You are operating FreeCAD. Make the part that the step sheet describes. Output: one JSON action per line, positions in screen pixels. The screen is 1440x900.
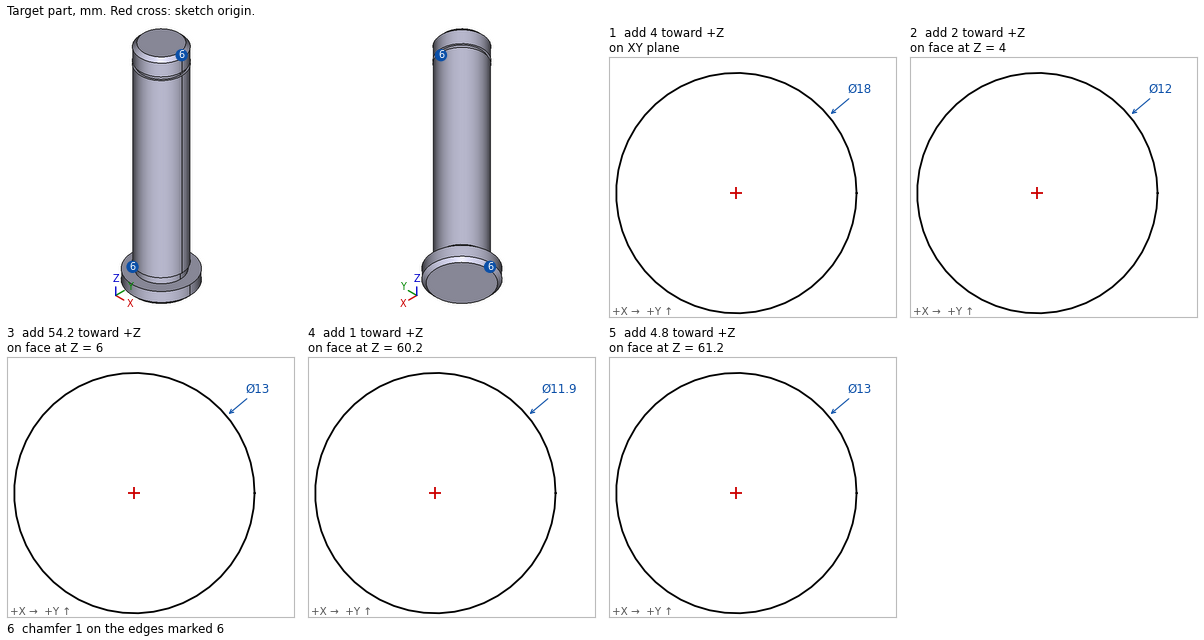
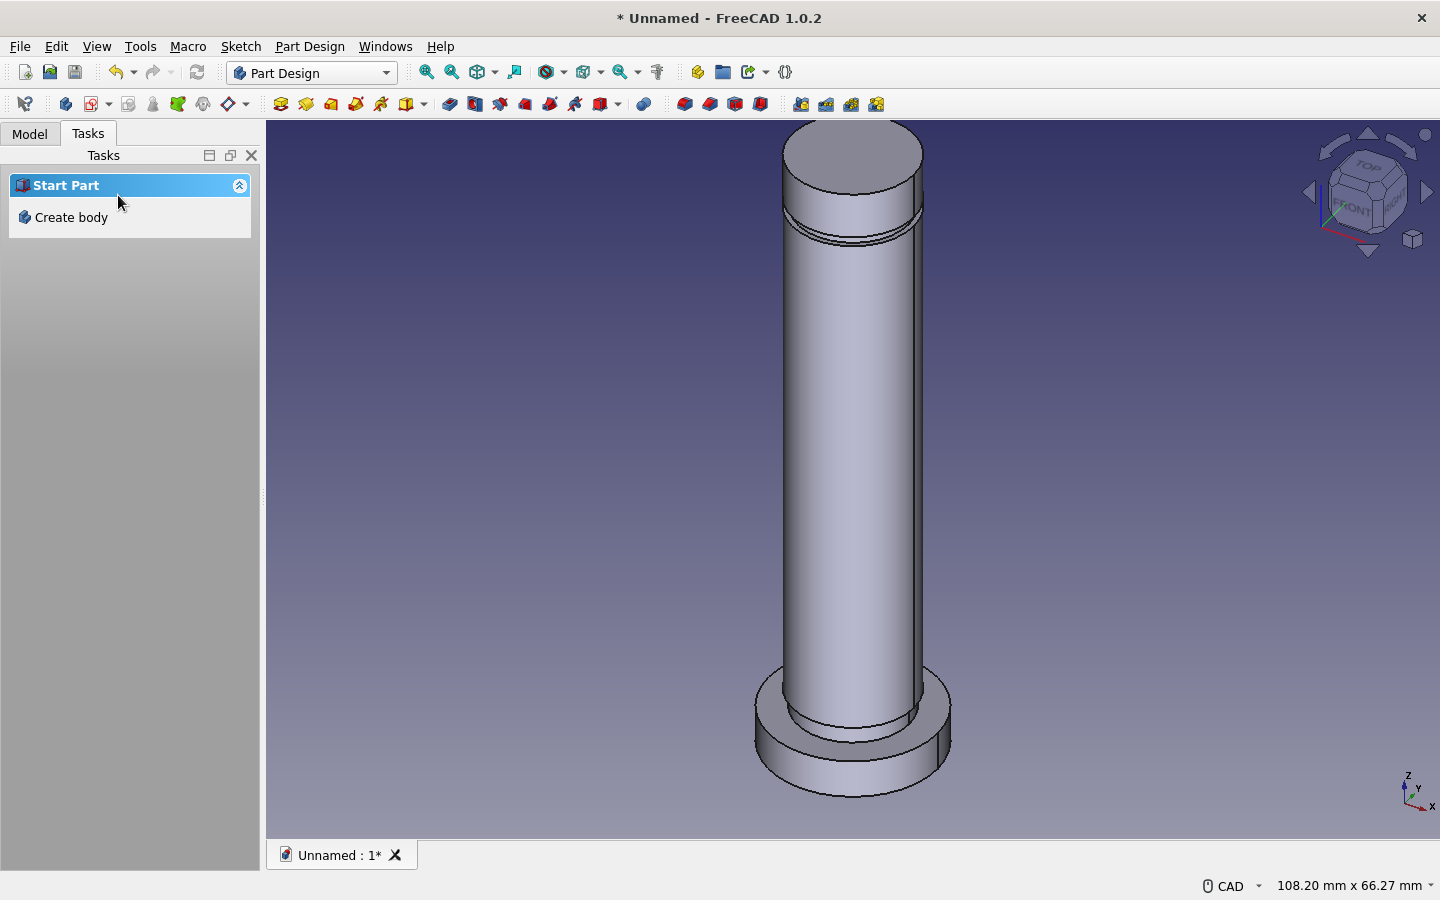
{"action": "left_click", "coordinate": [427, 72]}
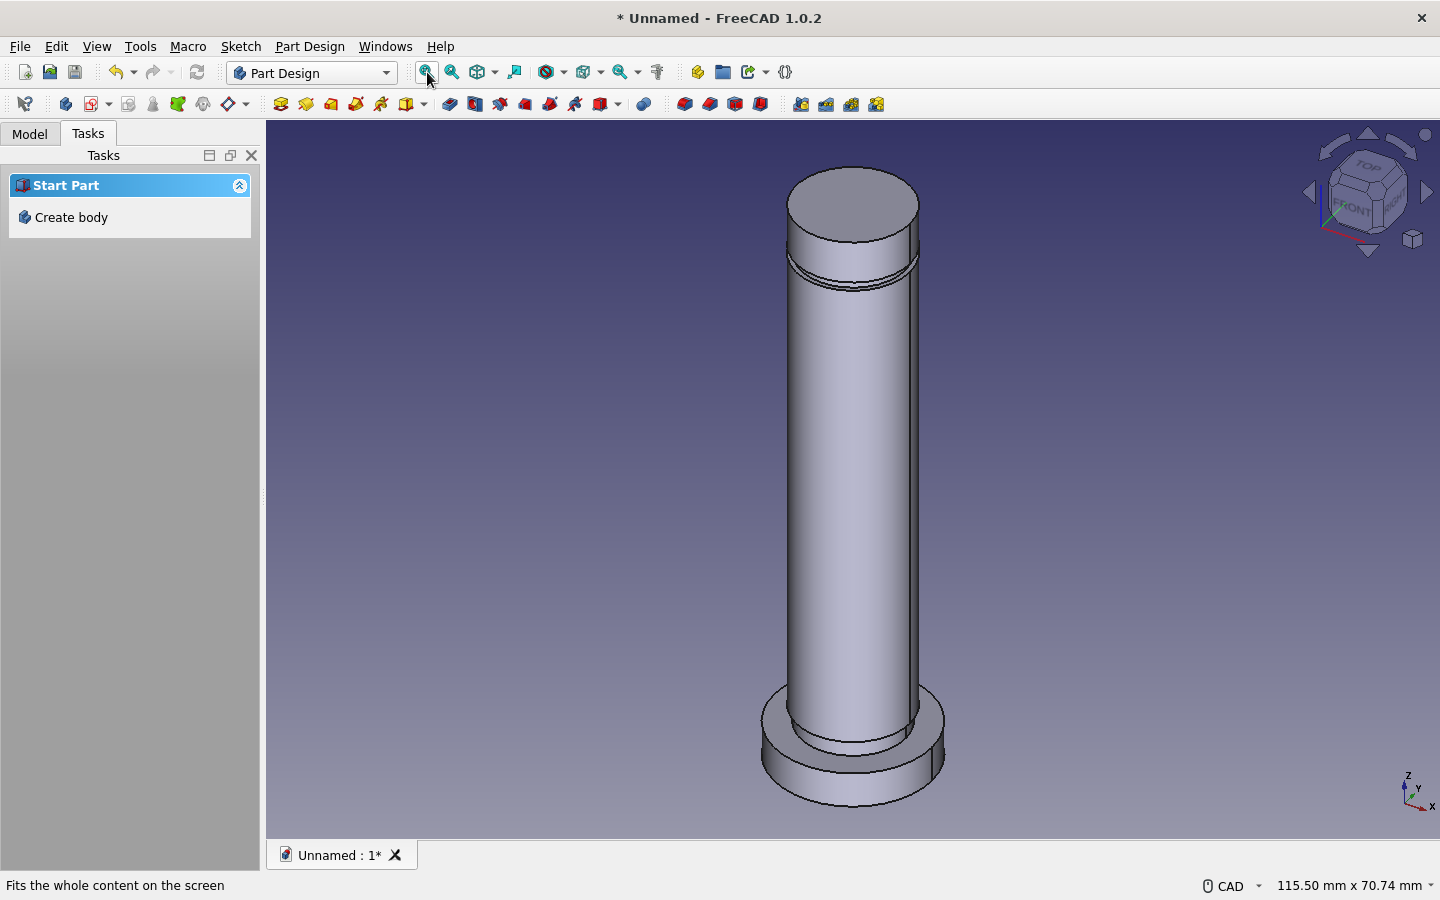
{"action": "left_click", "coordinate": [834, 805]}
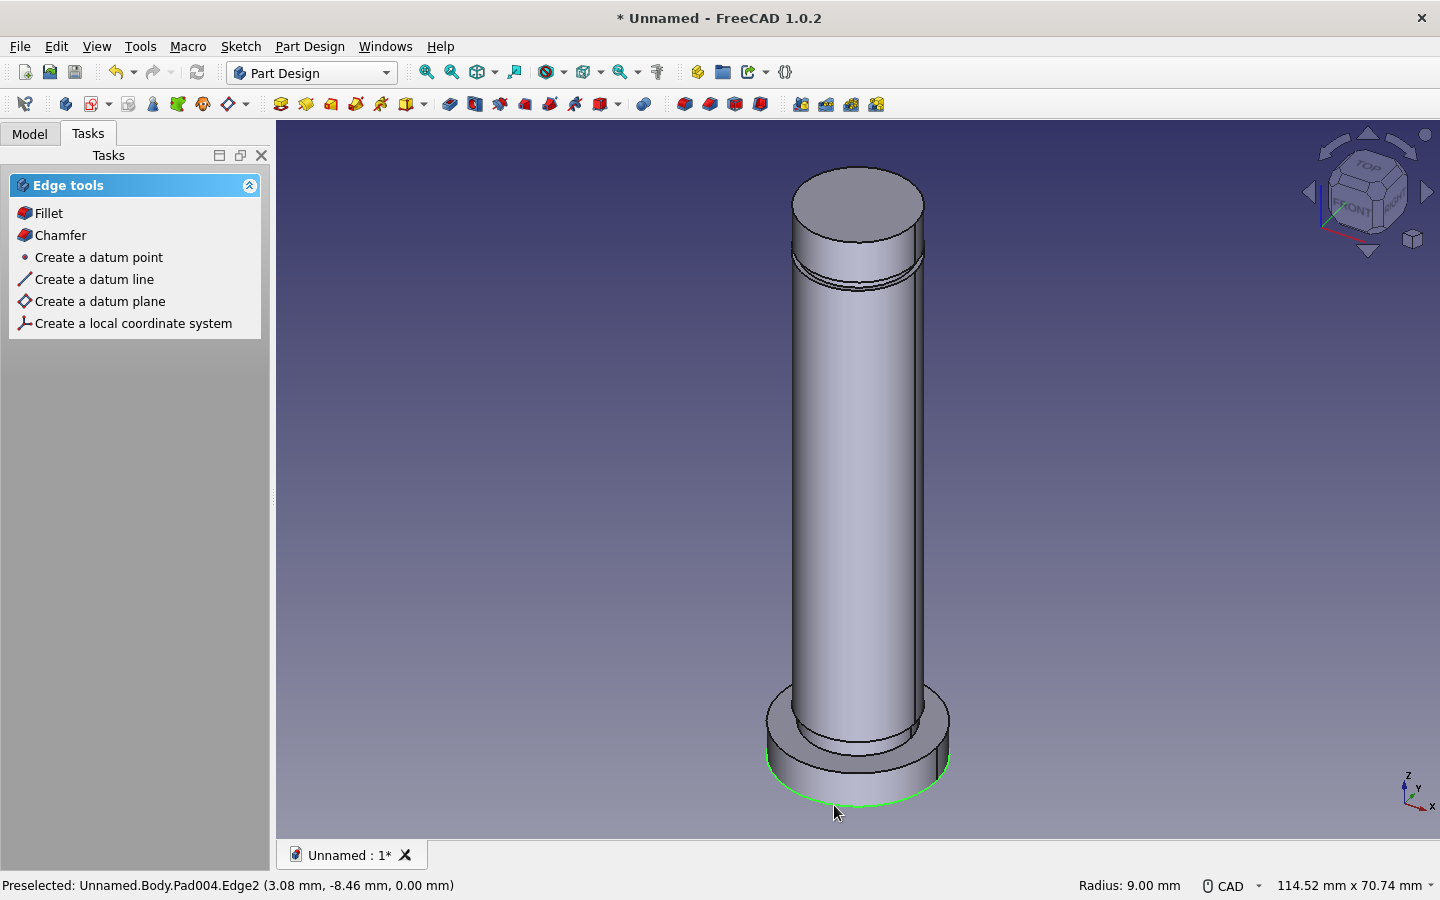
{"action": "left_click", "coordinate": [792, 208], "text": "ctrl"}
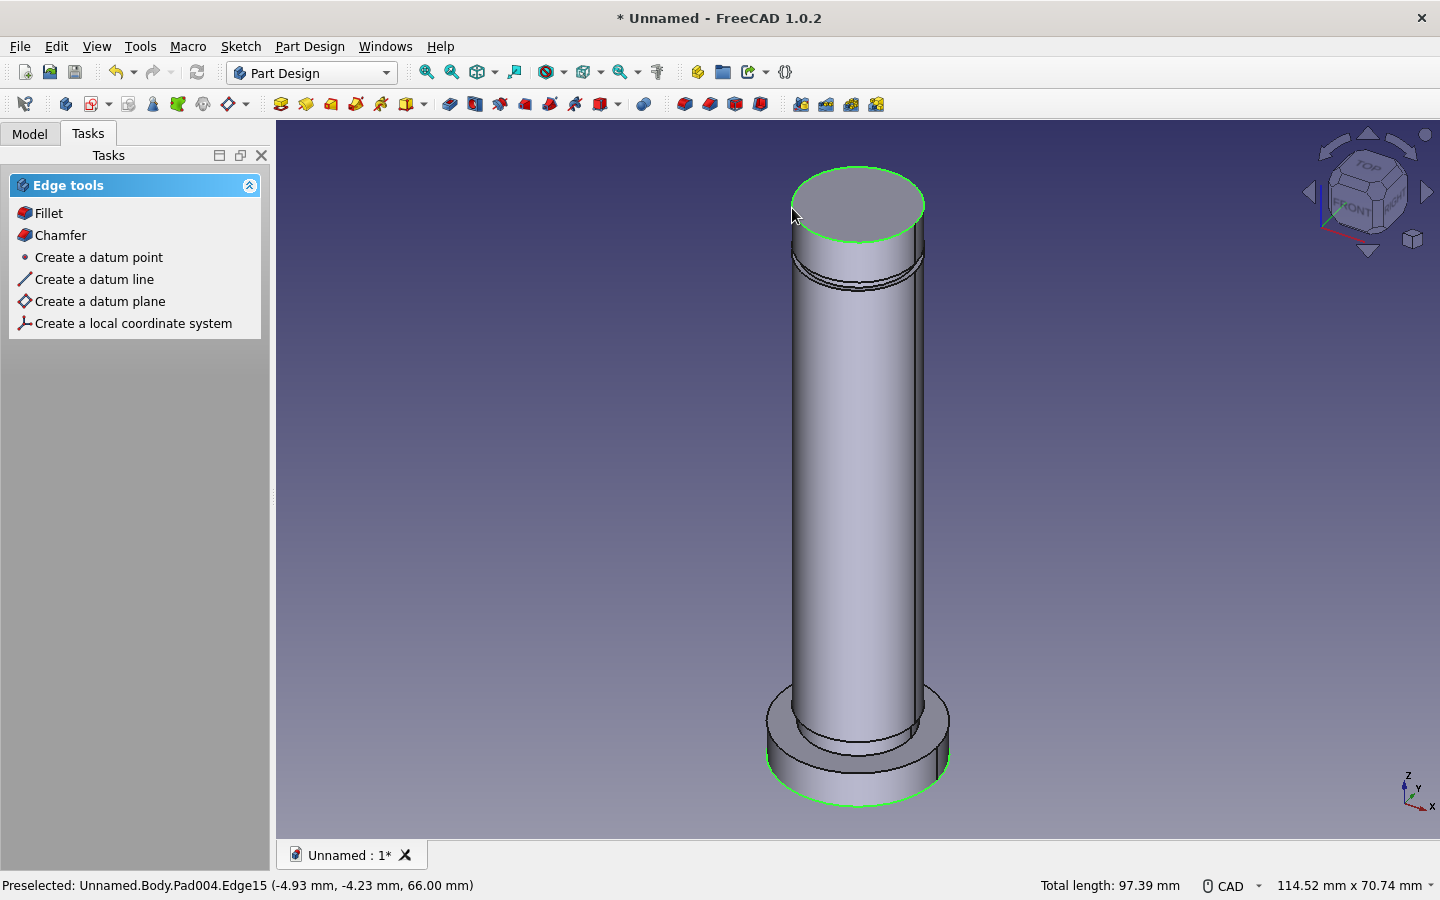
{"action": "left_click", "coordinate": [710, 104]}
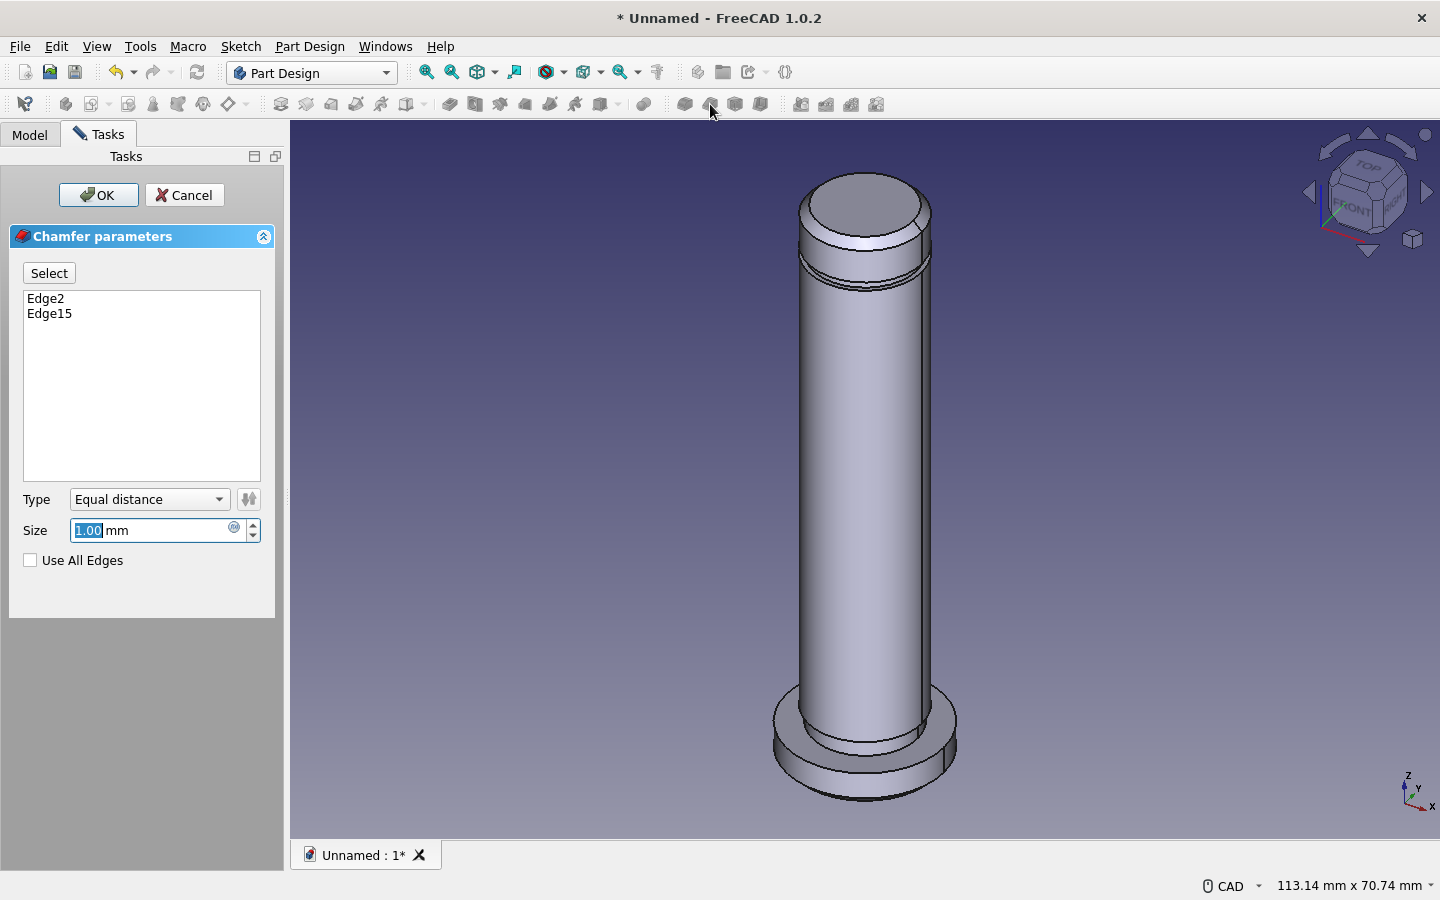
{"action": "type", "text": "1"}
{"action": "key", "text": "Tab"}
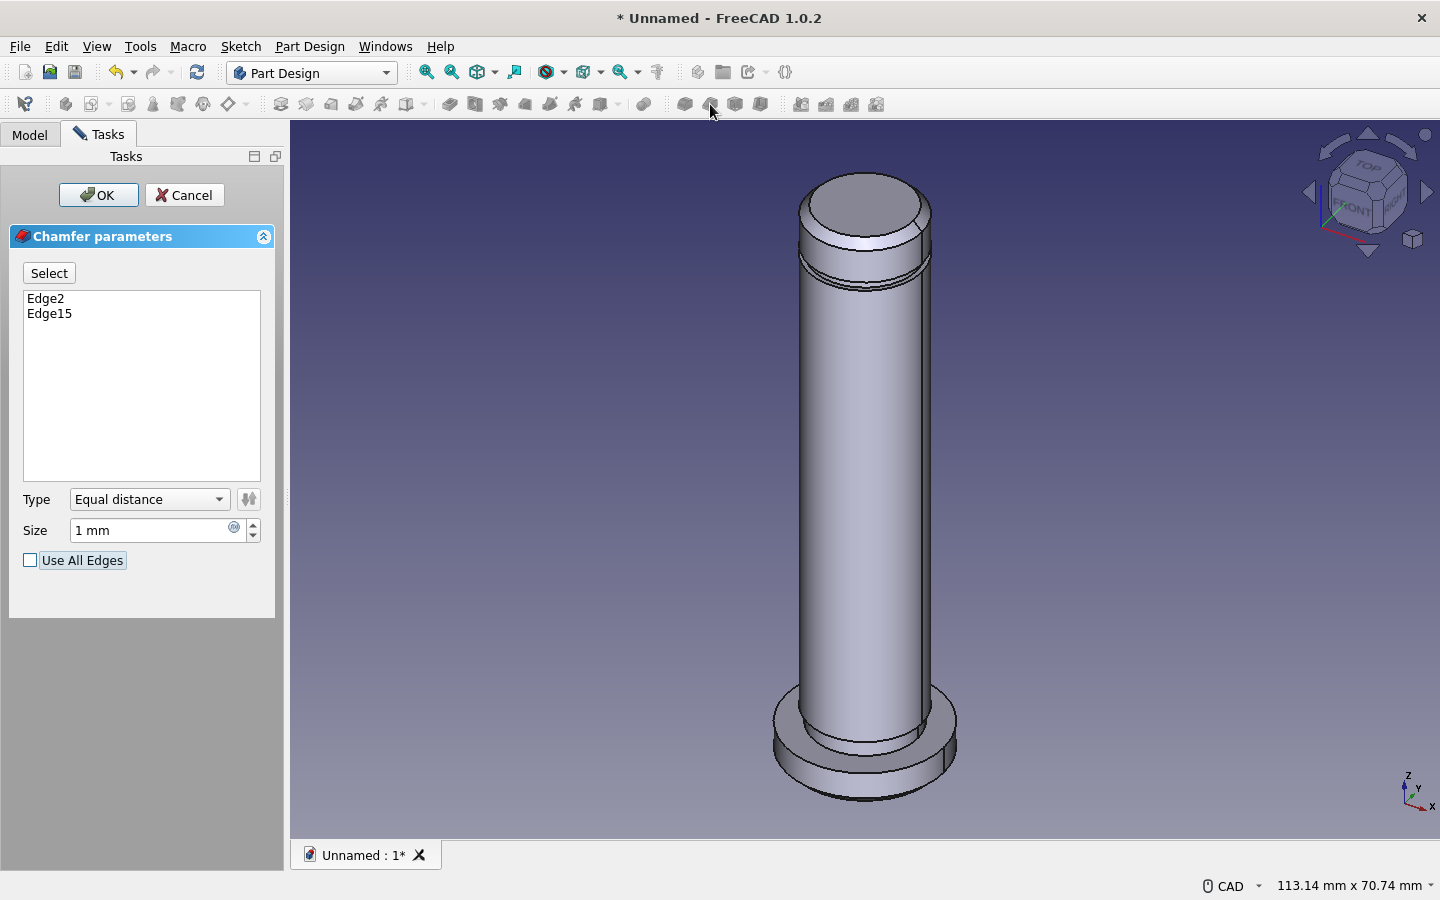
{"action": "left_click", "coordinate": [99, 195]}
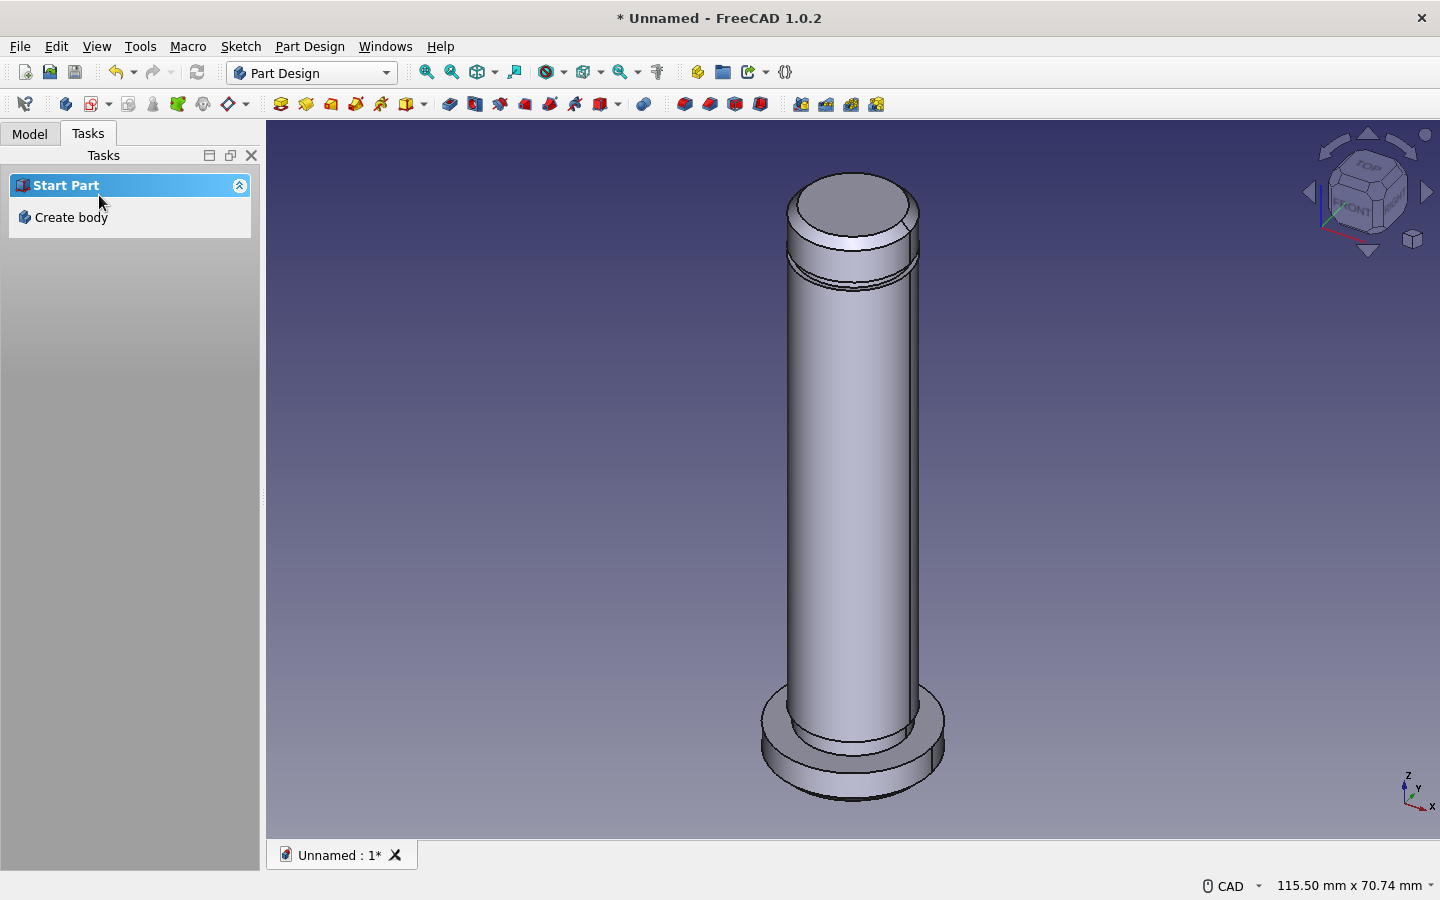
{"action": "key", "text": "0"}